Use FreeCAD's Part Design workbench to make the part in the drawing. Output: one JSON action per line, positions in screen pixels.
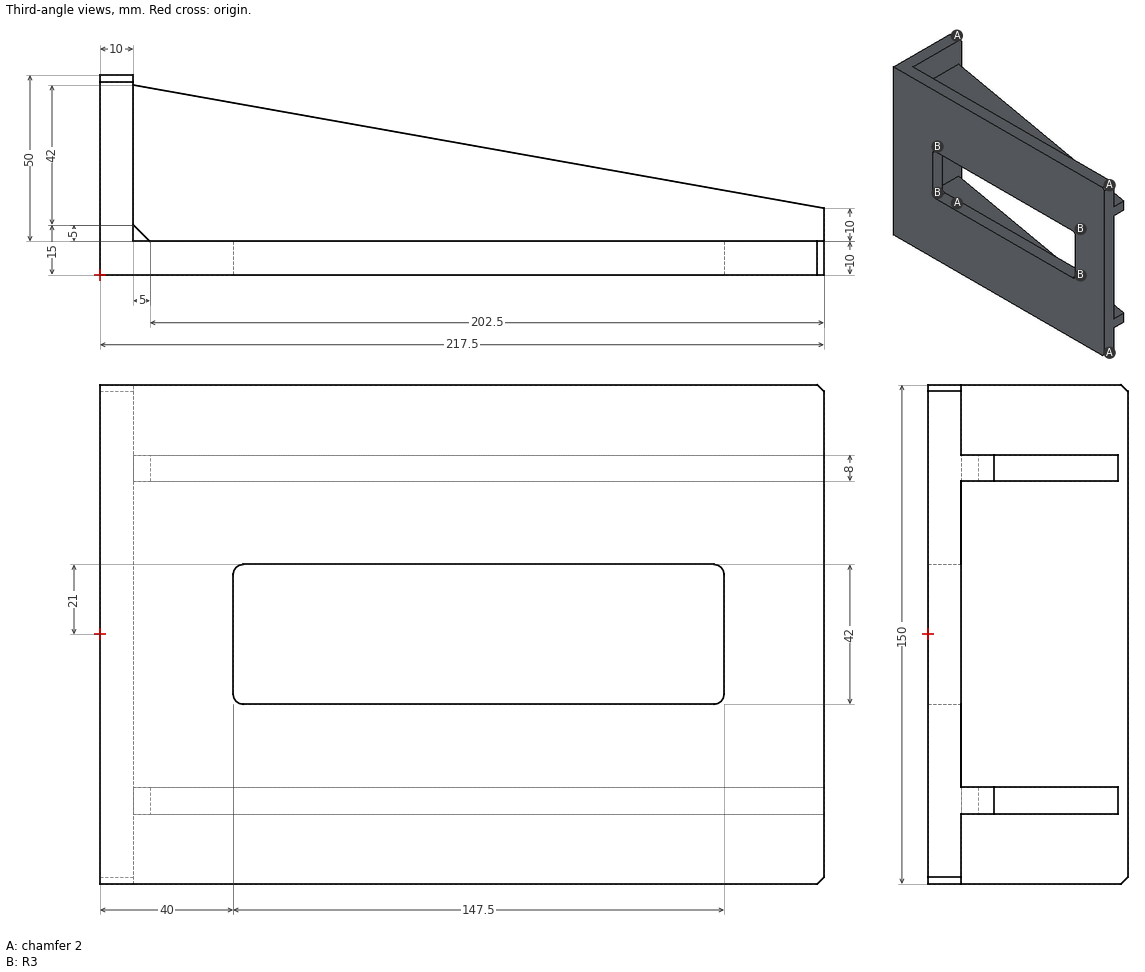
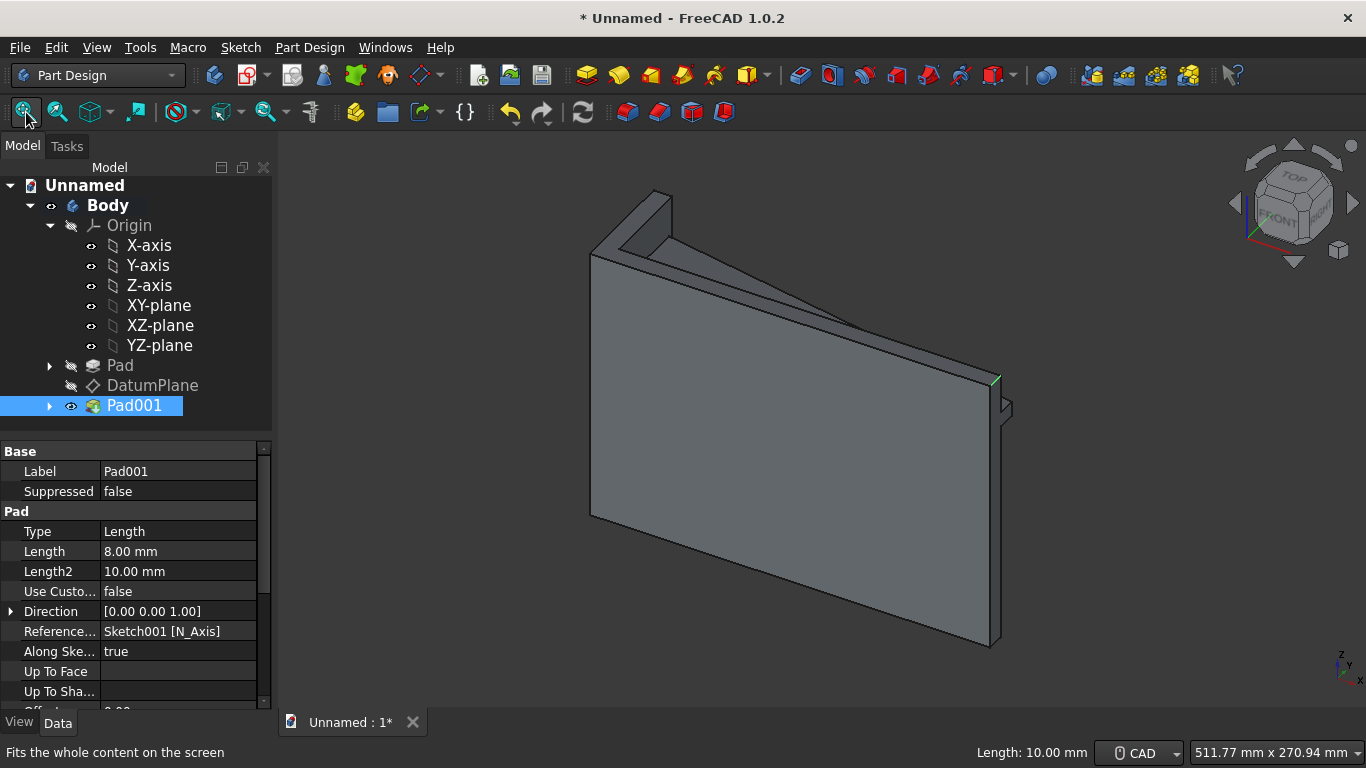
{"action": "key", "text": "0"}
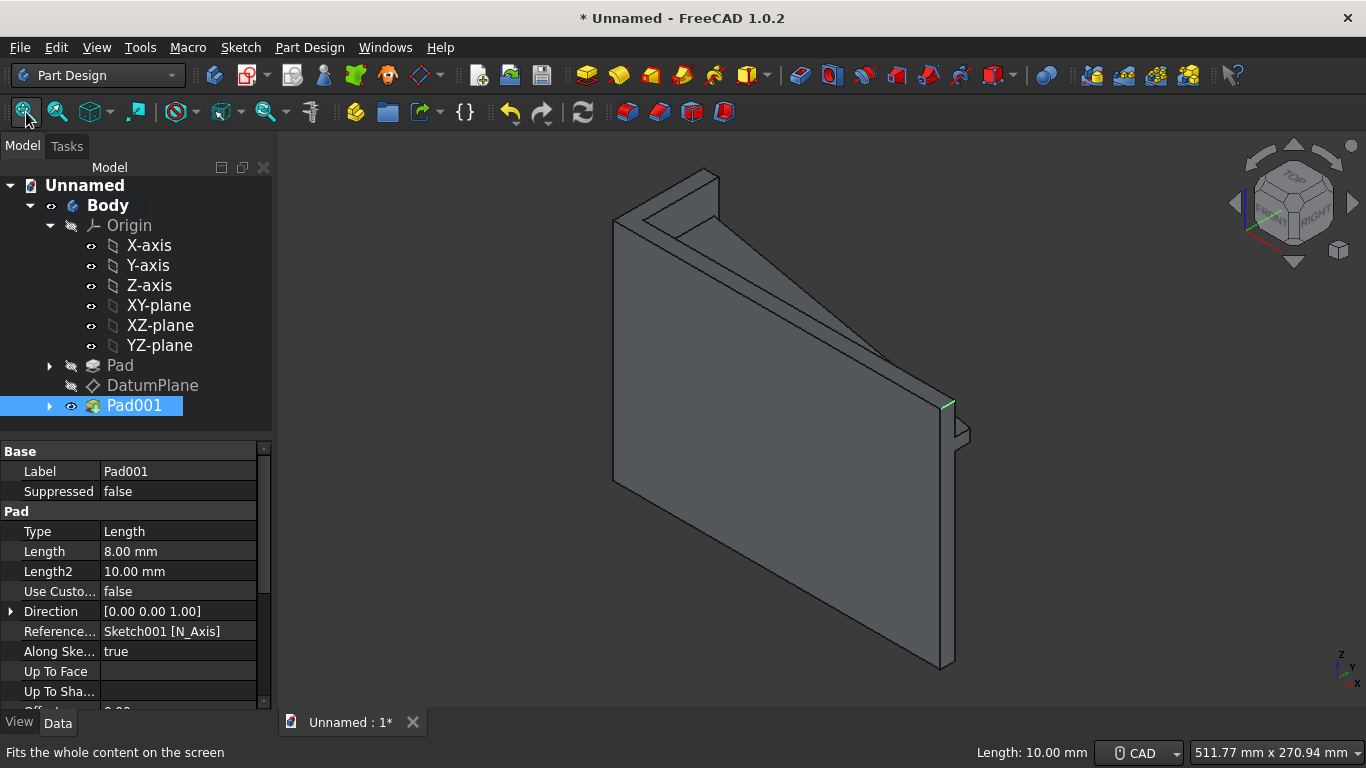
{"action": "scroll", "coordinate": [711, 172], "scroll_direction": "up", "scroll_amount": 4}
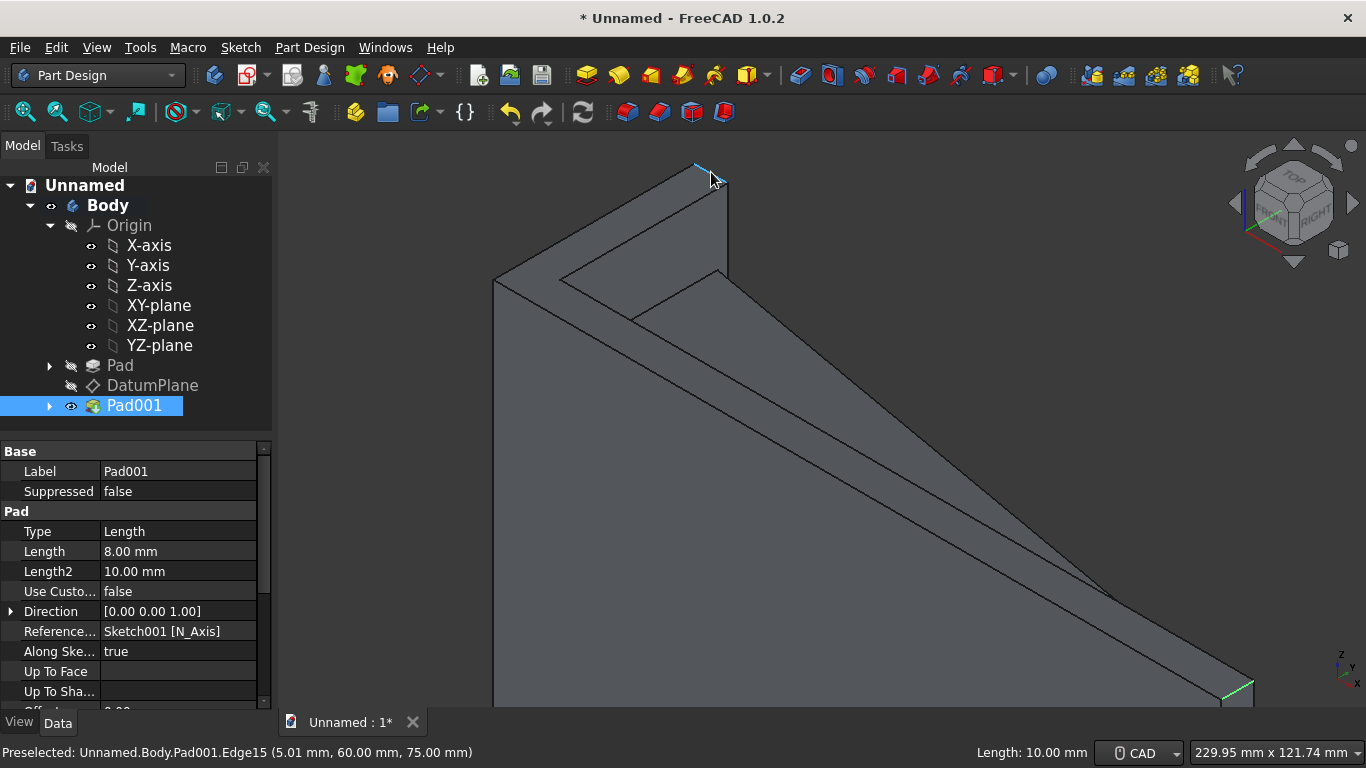
{"action": "left_click", "coordinate": [26, 112]}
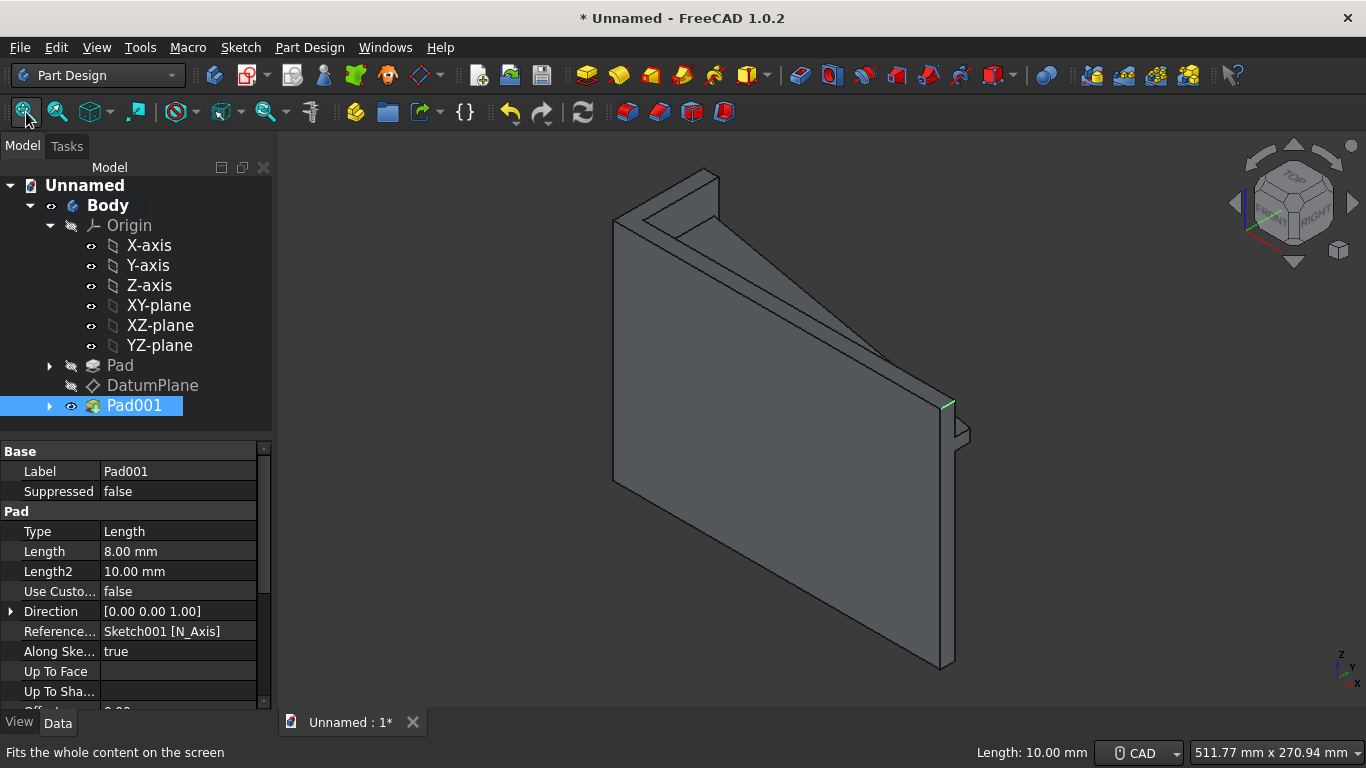
{"action": "key", "text": "2"}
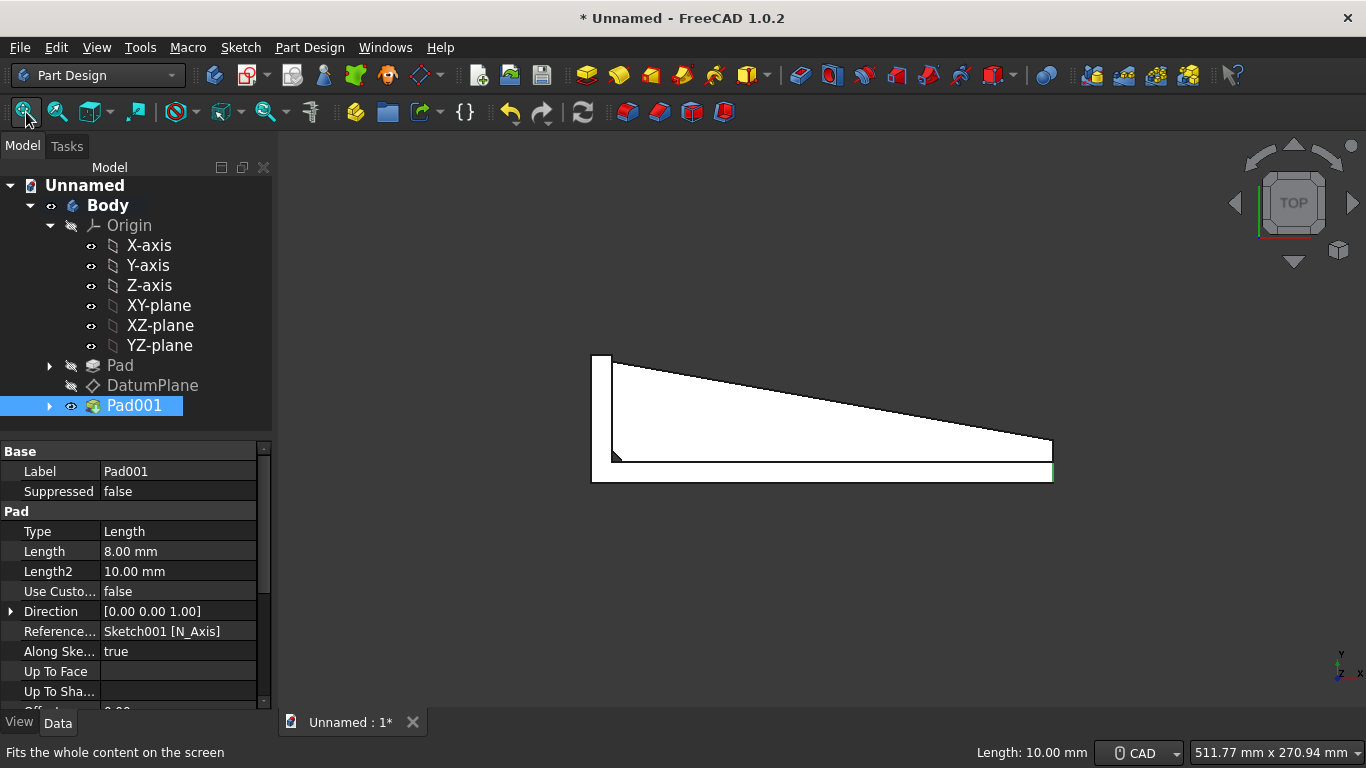
{"action": "left_click", "coordinate": [26, 112]}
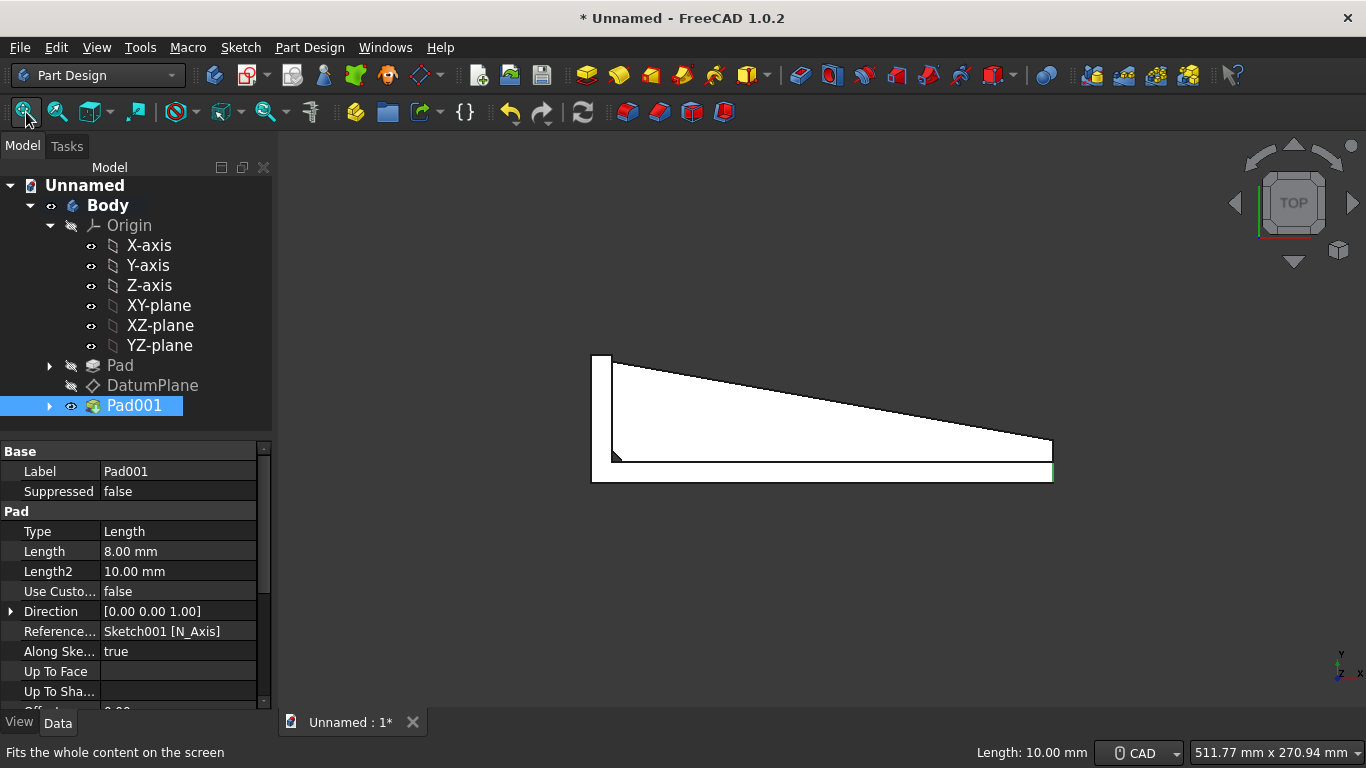
{"action": "left_click", "coordinate": [601, 354], "text": "ctrl"}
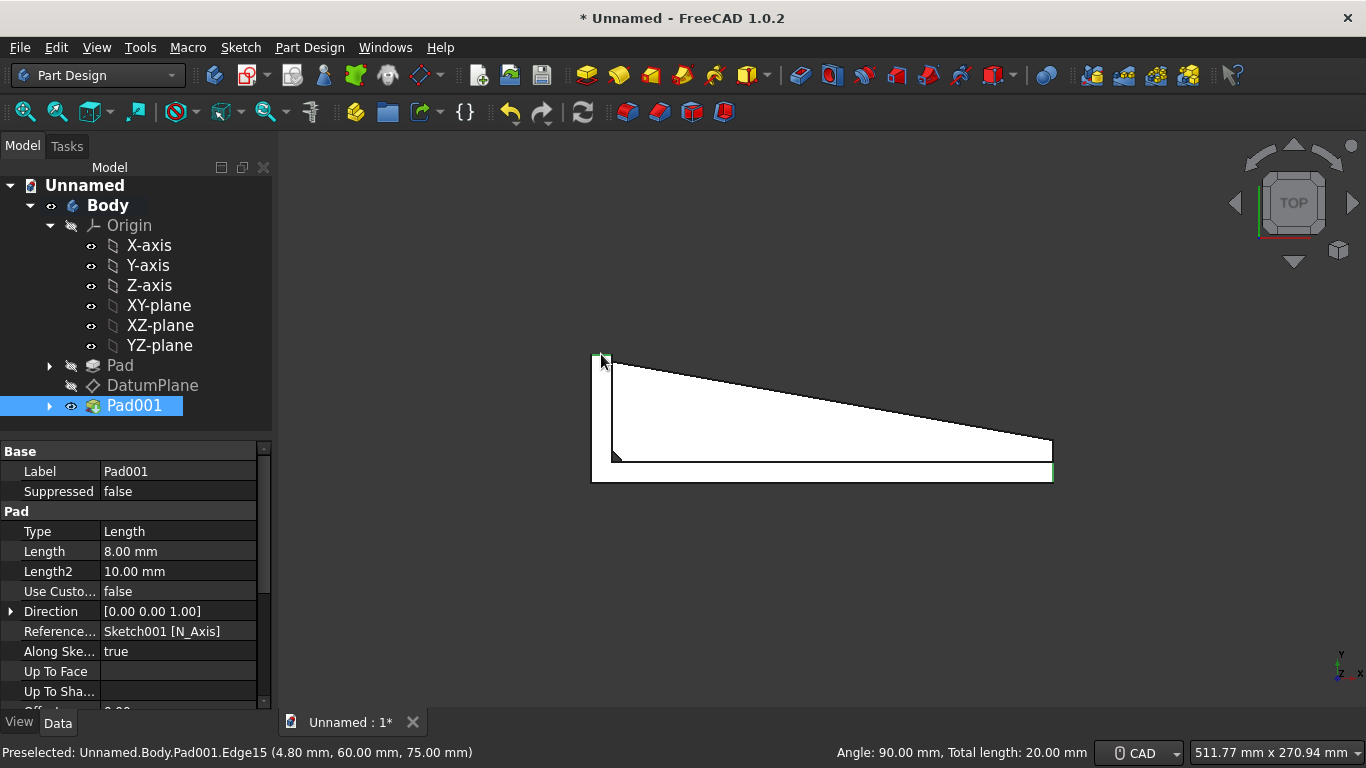
{"action": "scroll", "coordinate": [601, 354], "scroll_direction": "up", "scroll_amount": 4}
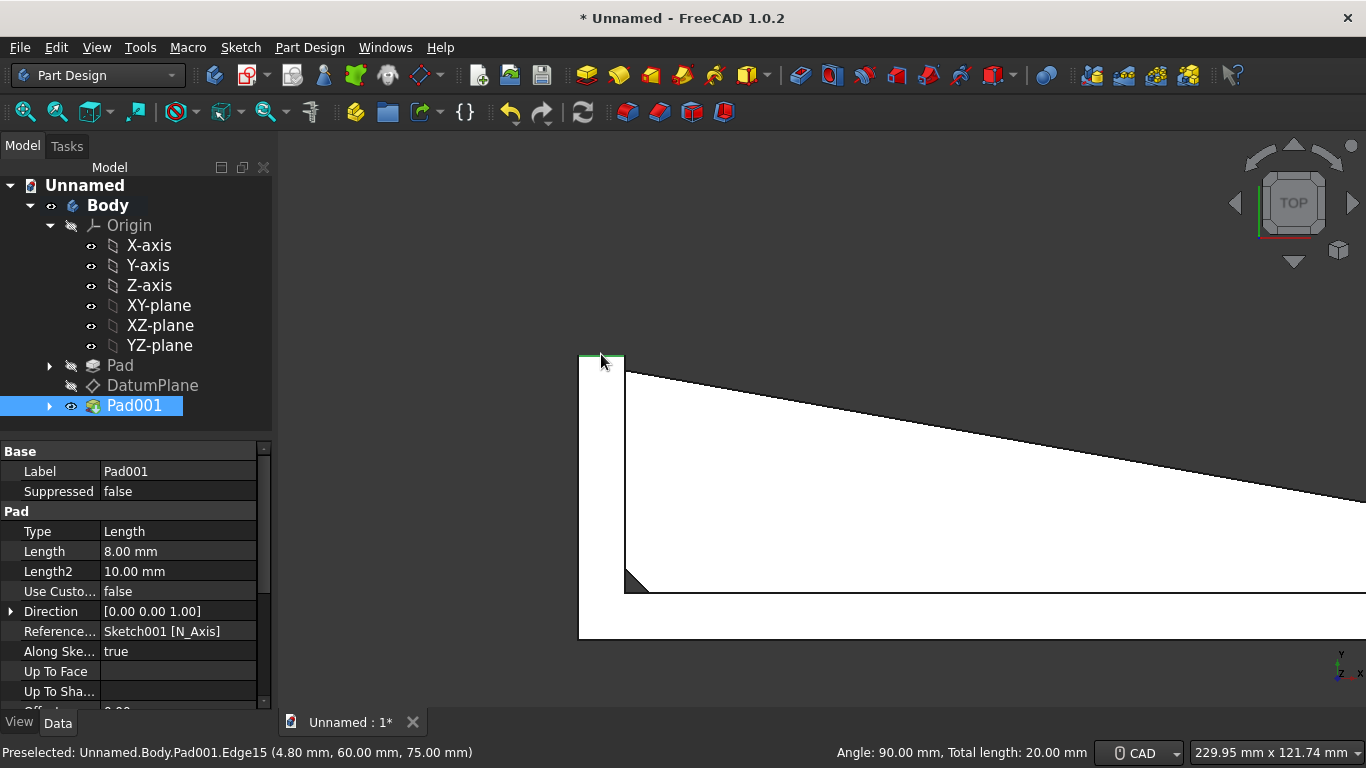
{"action": "left_click", "coordinate": [26, 112]}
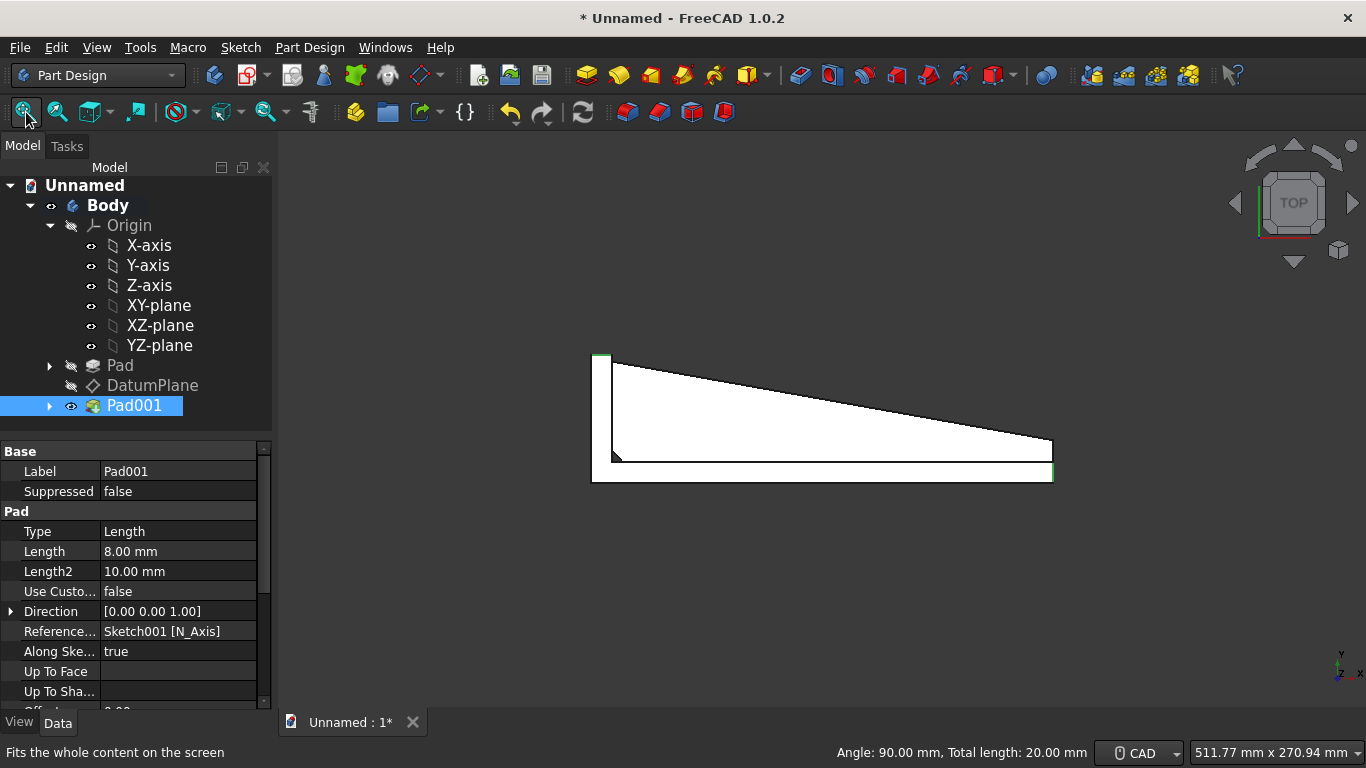
{"action": "key", "text": "1"}